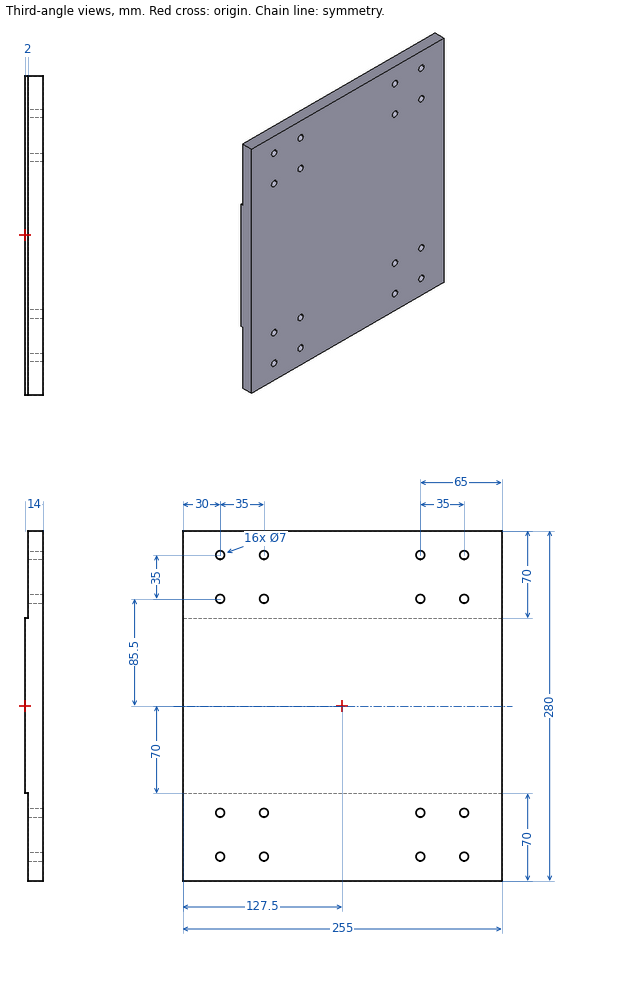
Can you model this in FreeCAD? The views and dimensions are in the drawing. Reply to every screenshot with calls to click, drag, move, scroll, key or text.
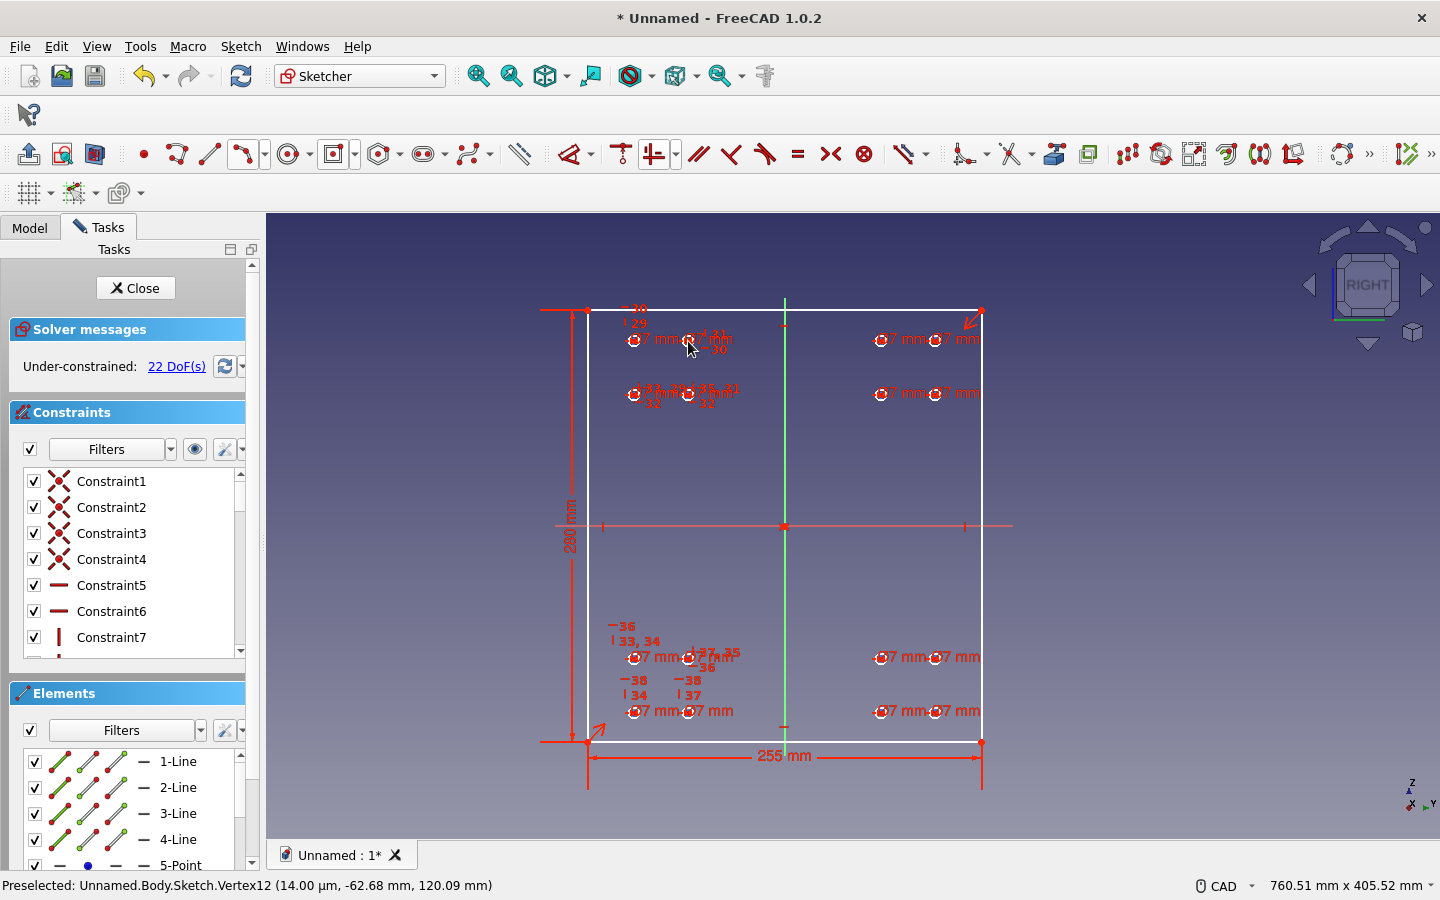
click(881, 341)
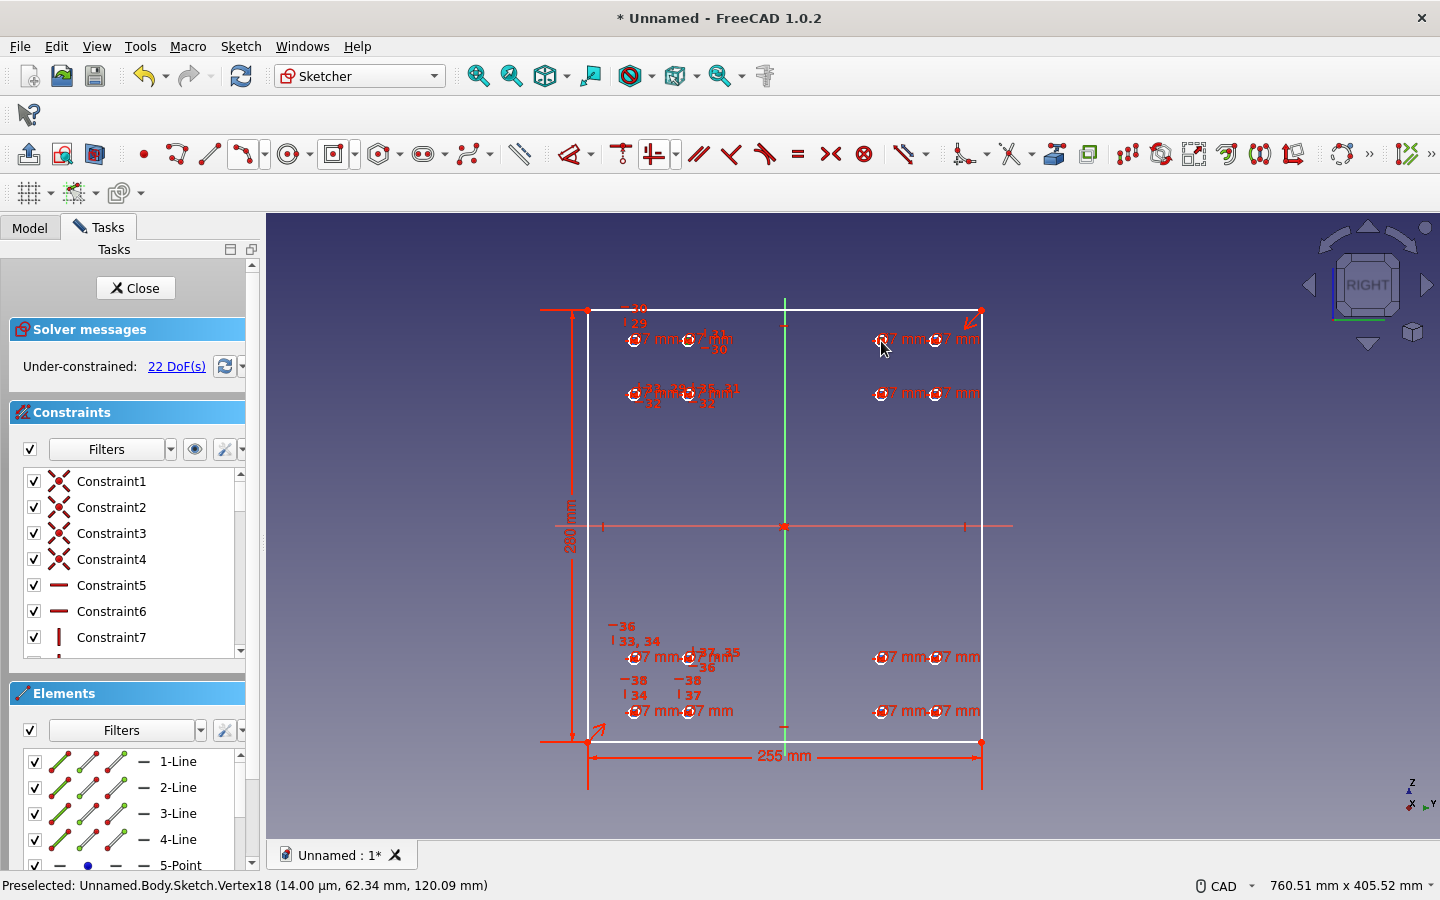
click(676, 154)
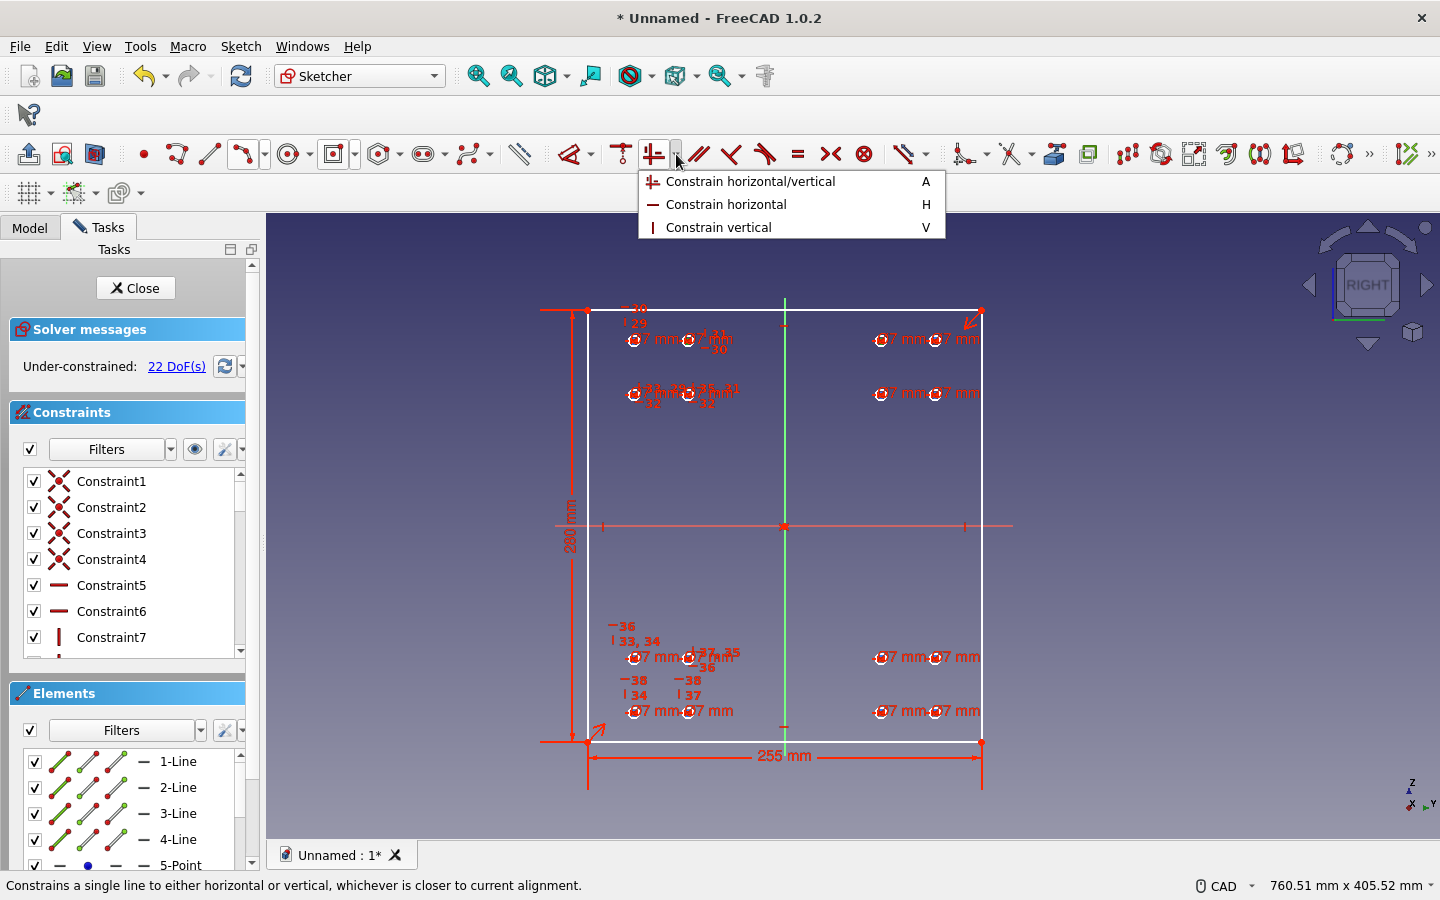
click(792, 204)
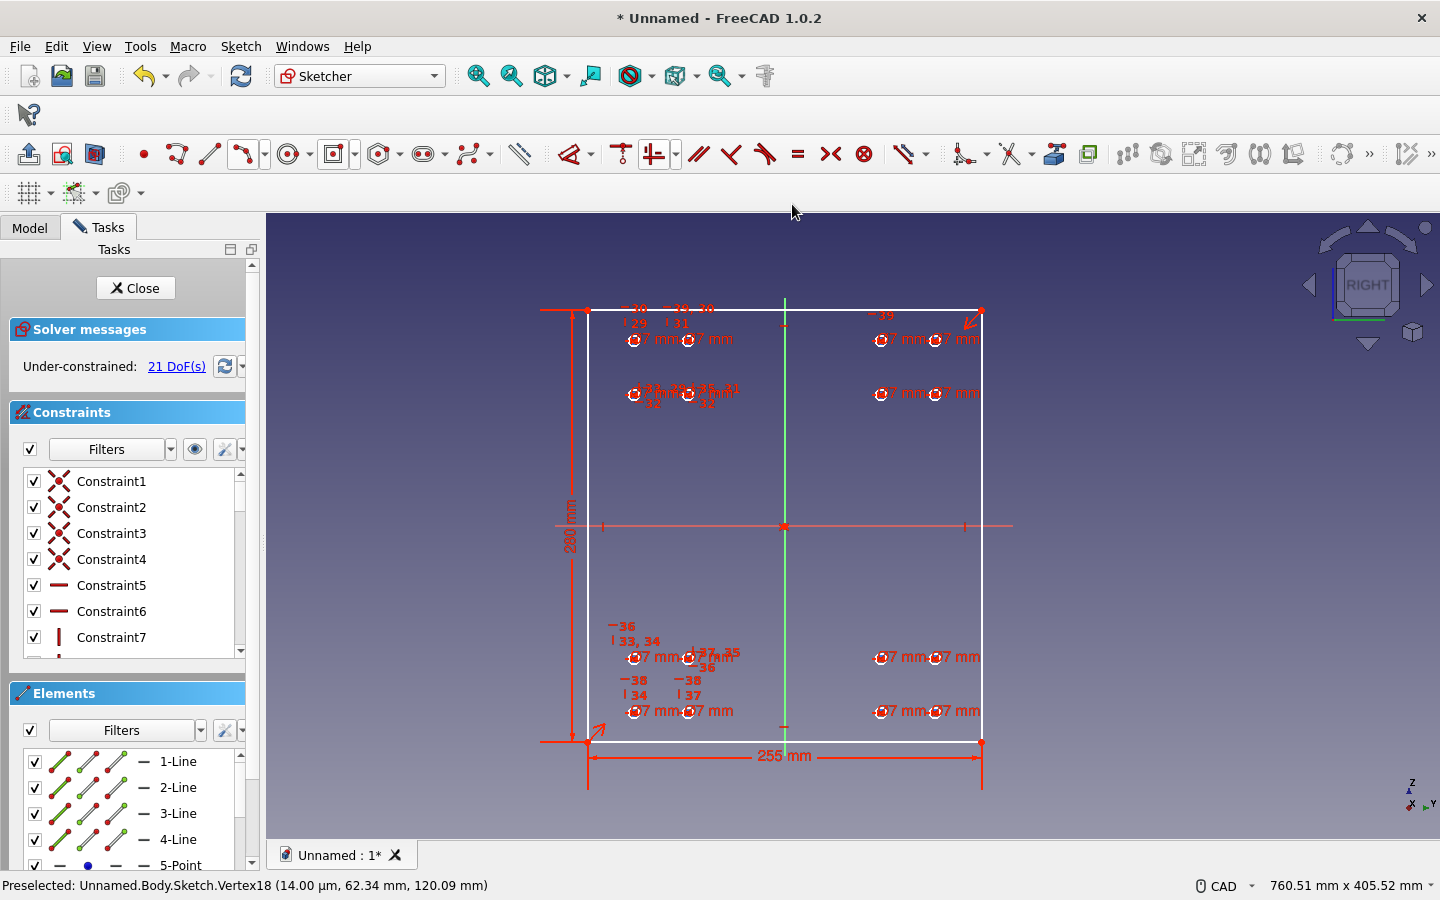
click(881, 341)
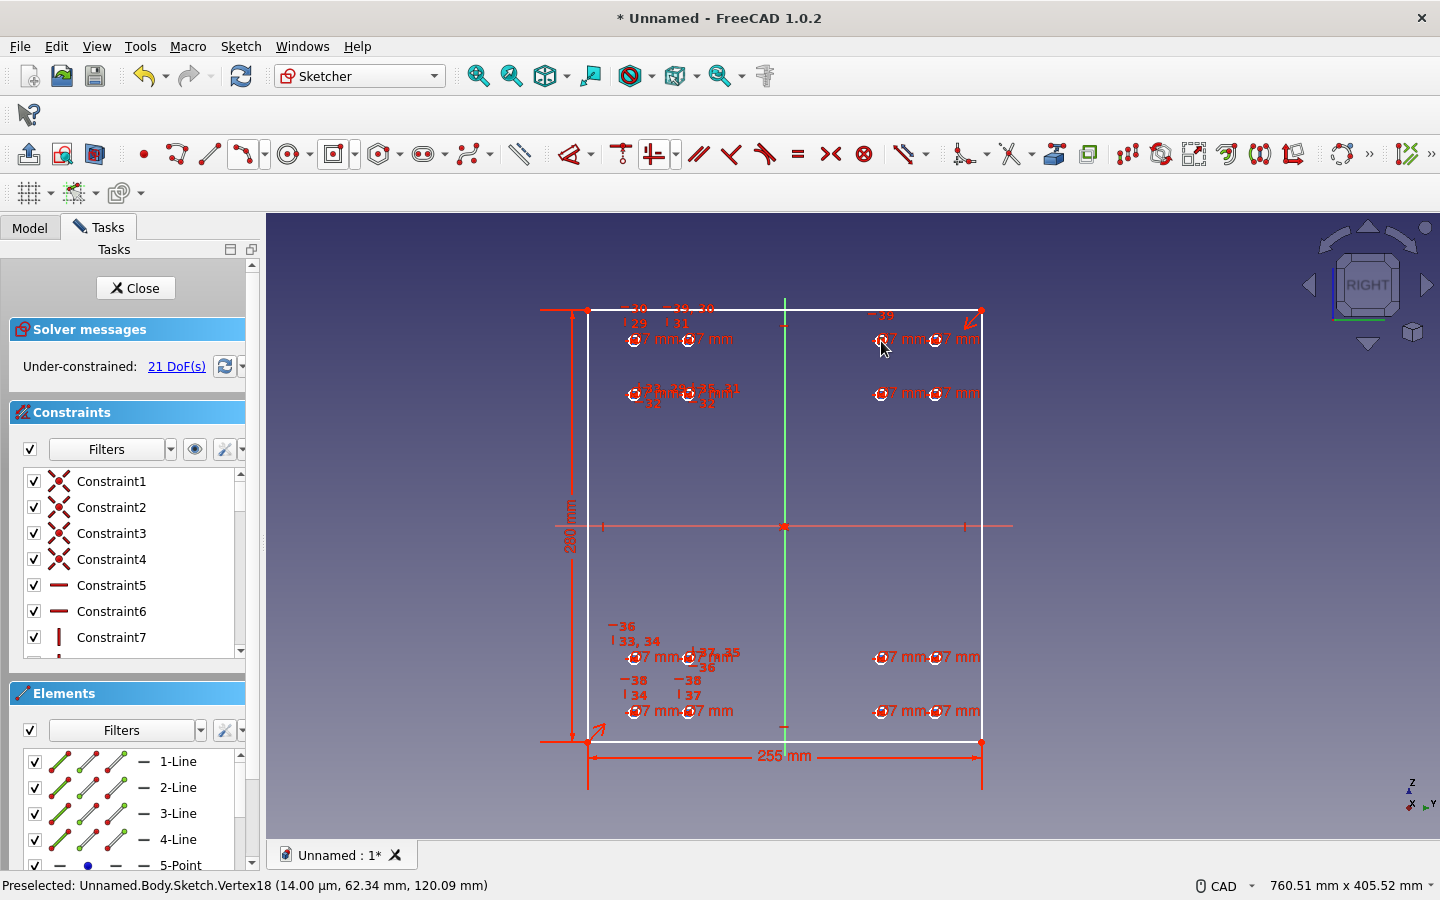
click(881, 395)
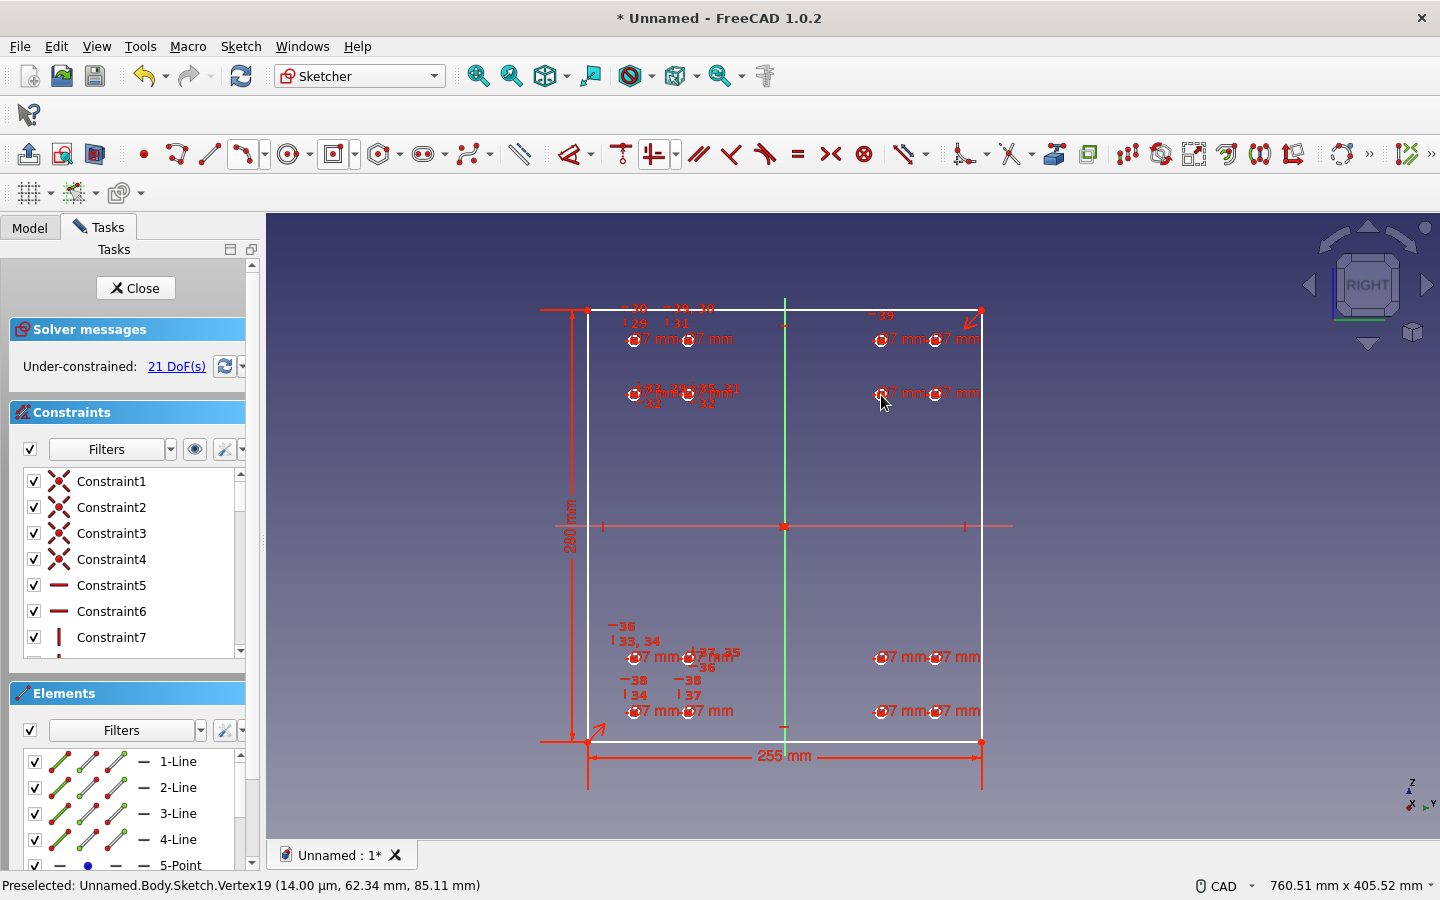
click(676, 154)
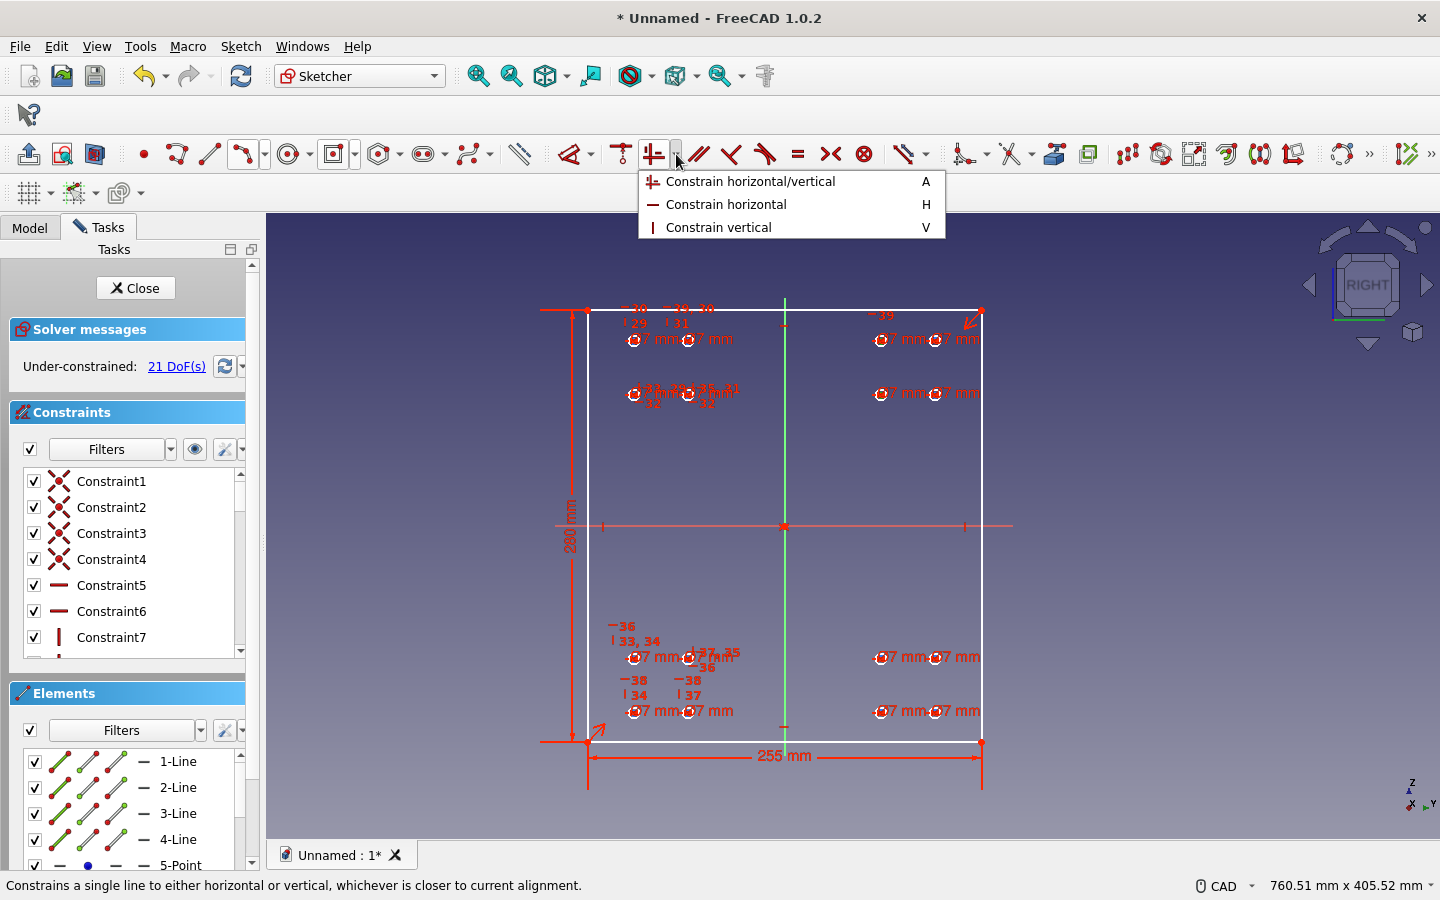
click(792, 228)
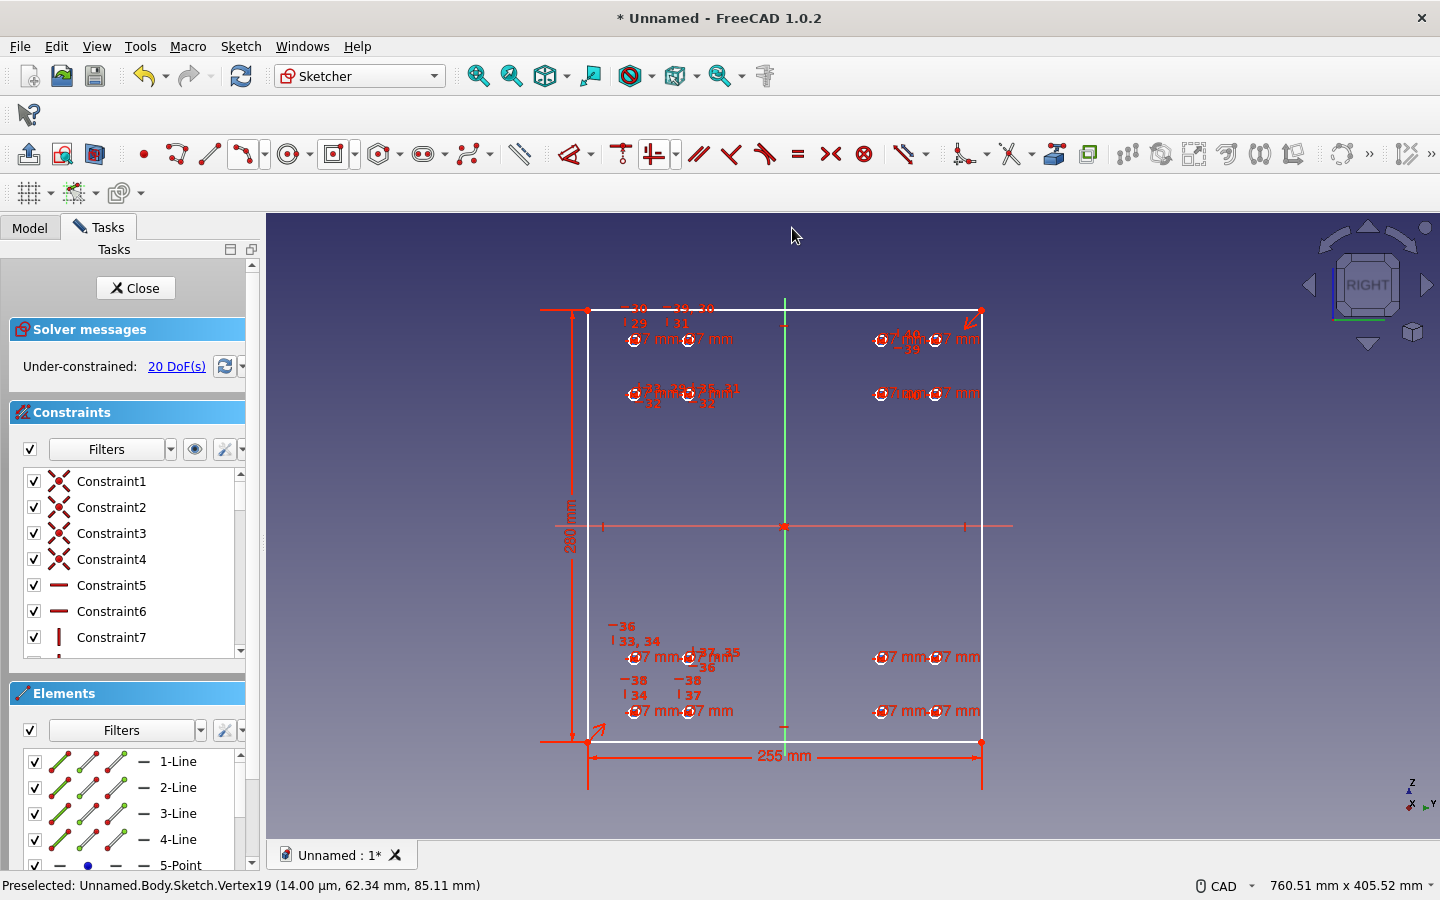
click(688, 395)